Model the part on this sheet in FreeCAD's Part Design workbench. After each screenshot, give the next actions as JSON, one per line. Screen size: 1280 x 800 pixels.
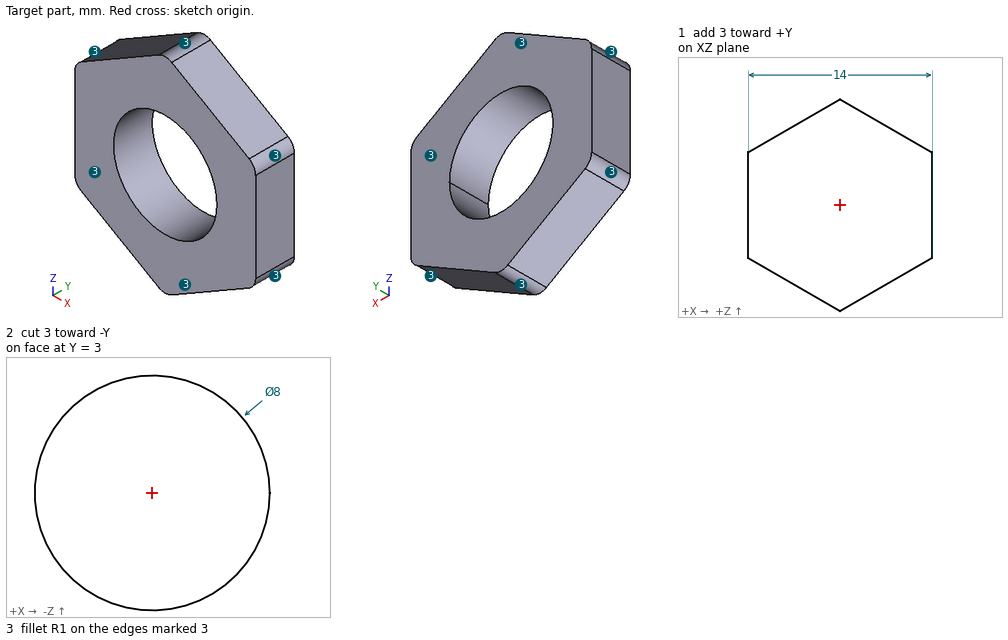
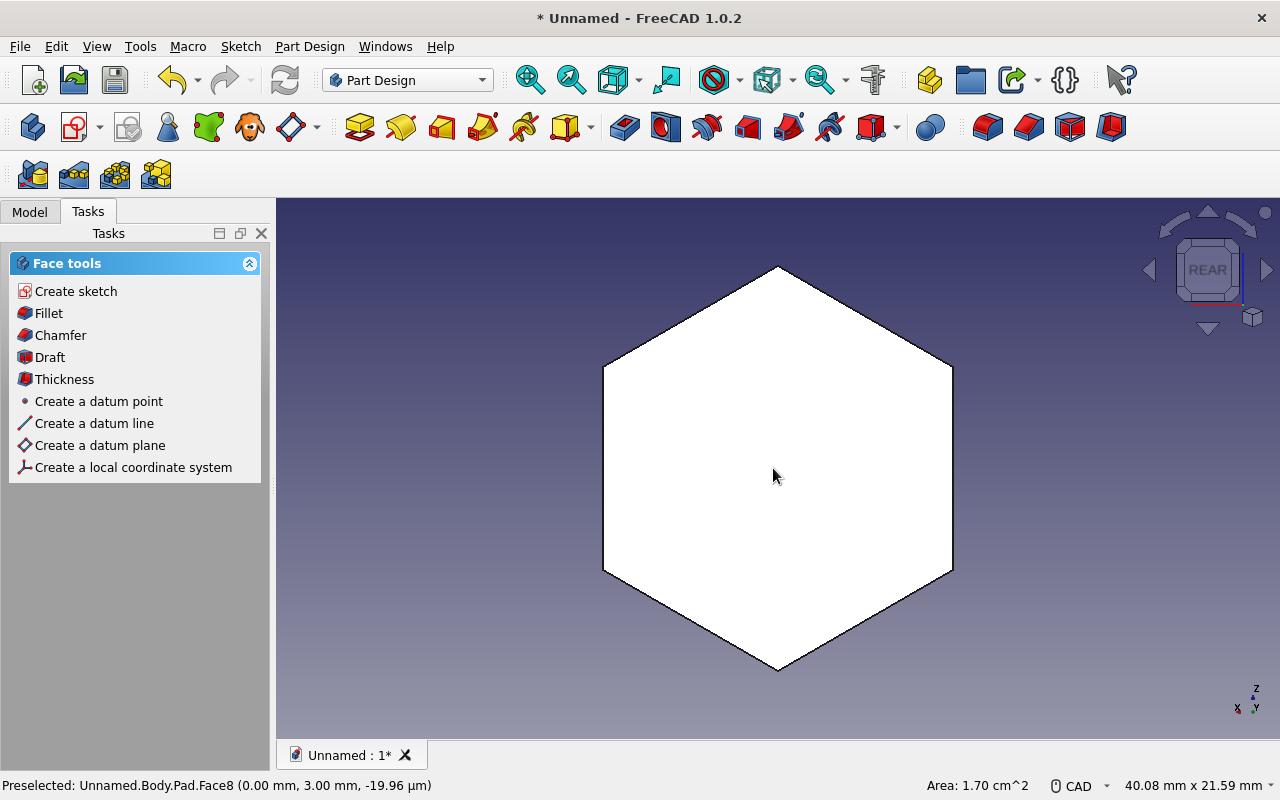
{"action": "left_click", "coordinate": [74, 128]}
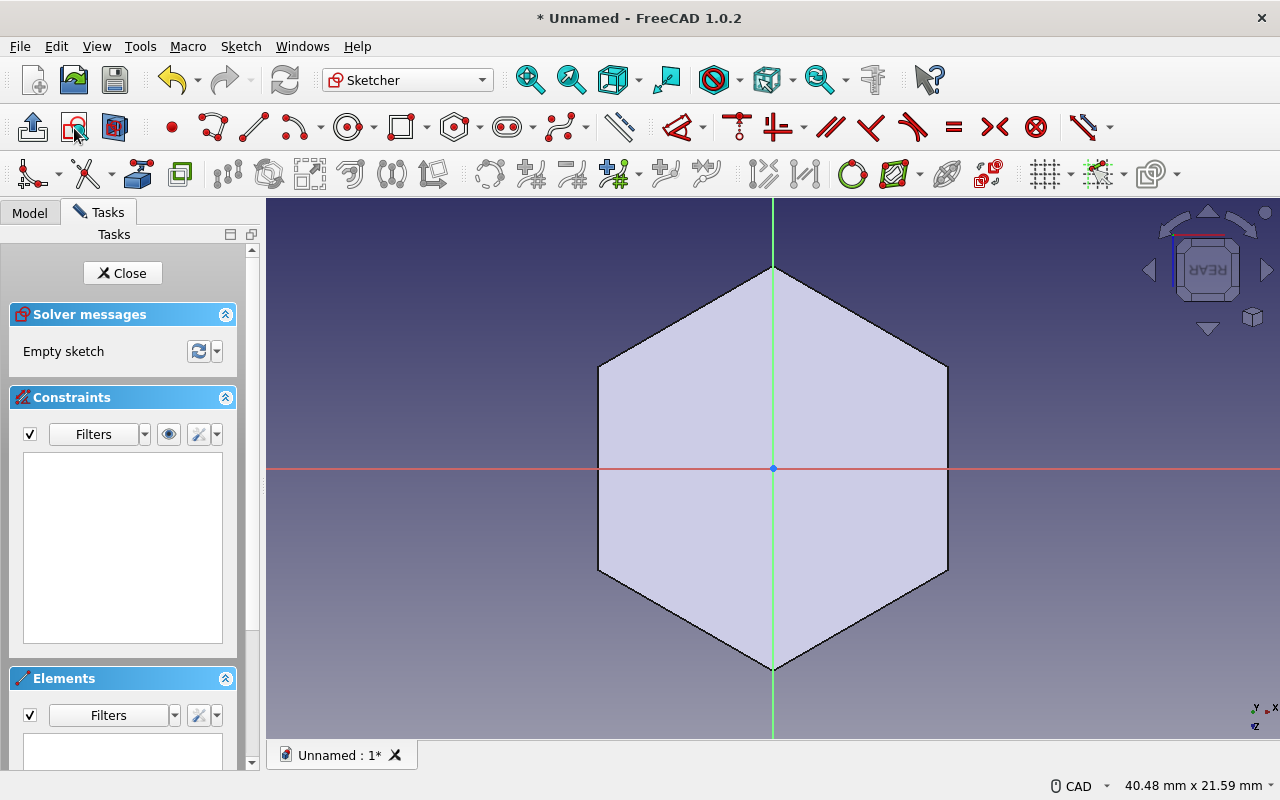
{"action": "scroll", "coordinate": [856, 468], "scroll_direction": "up", "scroll_amount": 3}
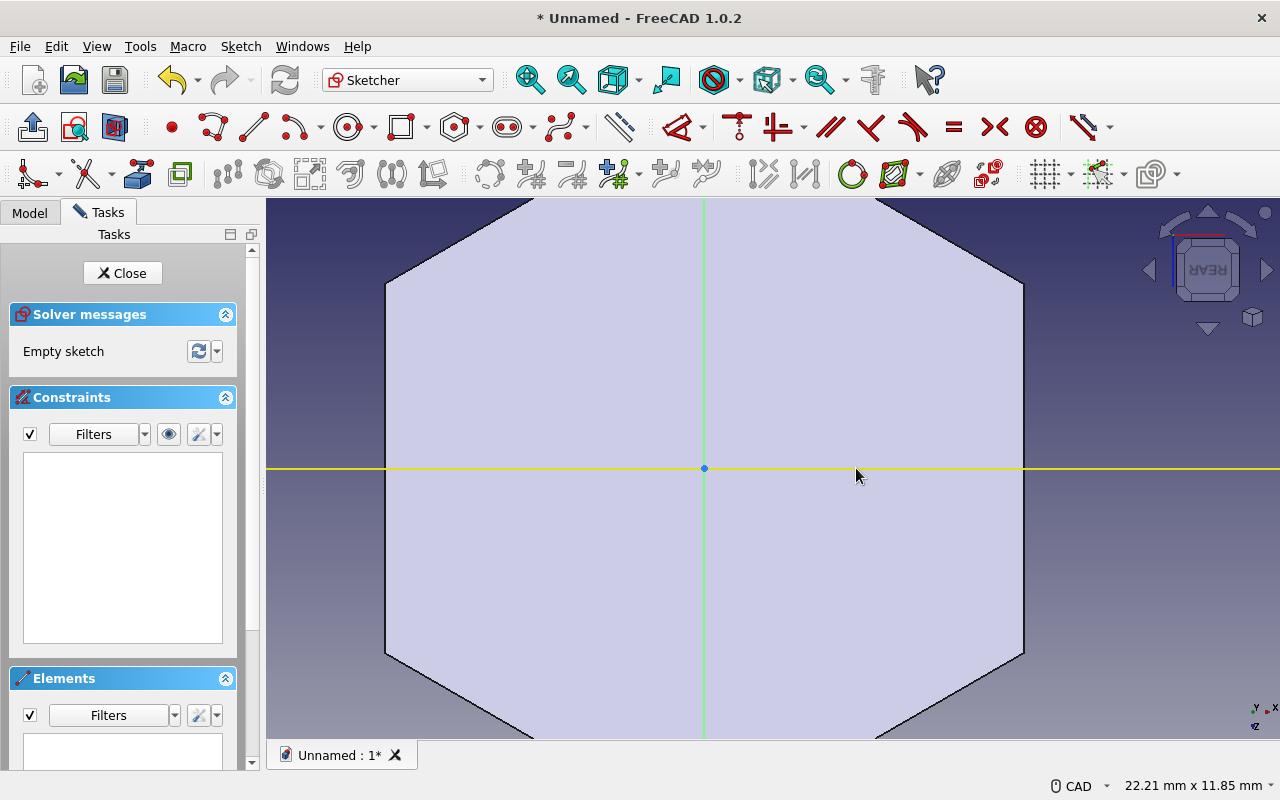
{"action": "key", "text": "g c"}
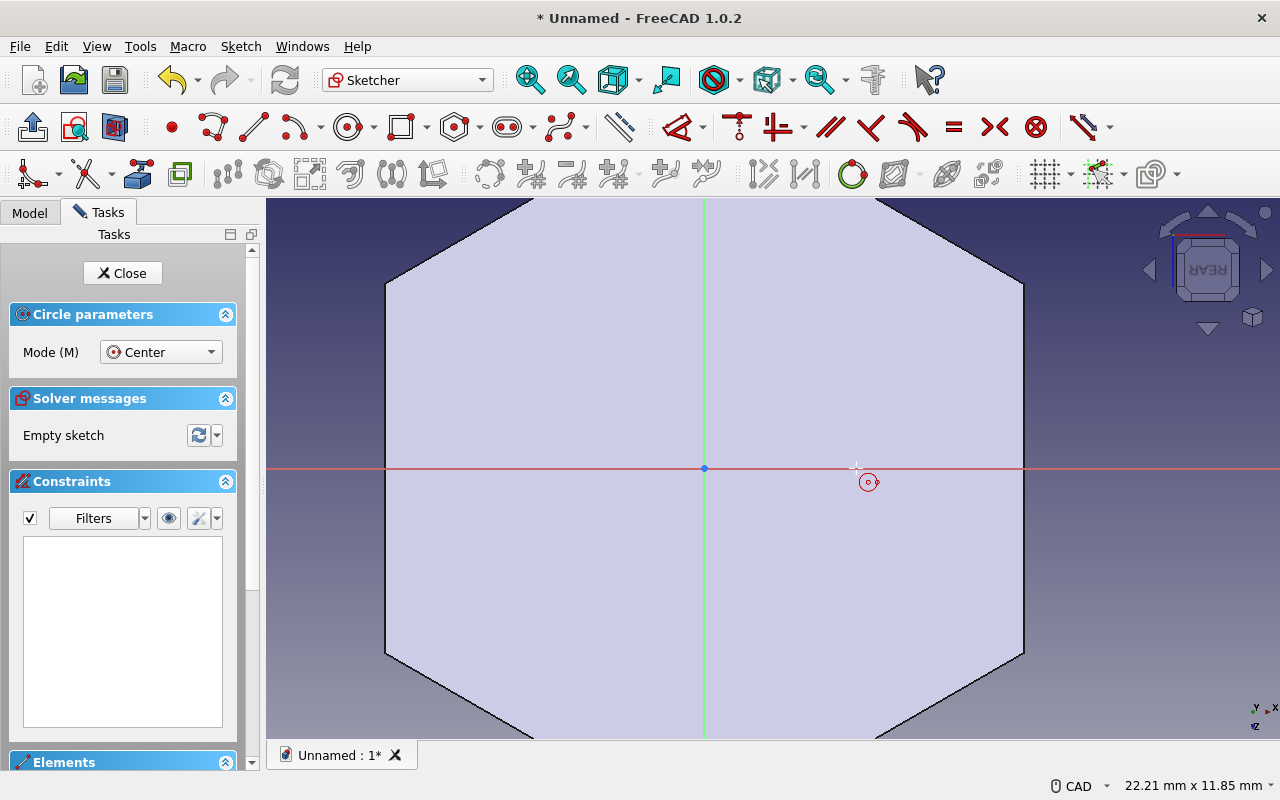
{"action": "left_click", "coordinate": [704, 468]}
{"action": "left_click", "coordinate": [833, 339]}
{"action": "key", "text": "Escape"}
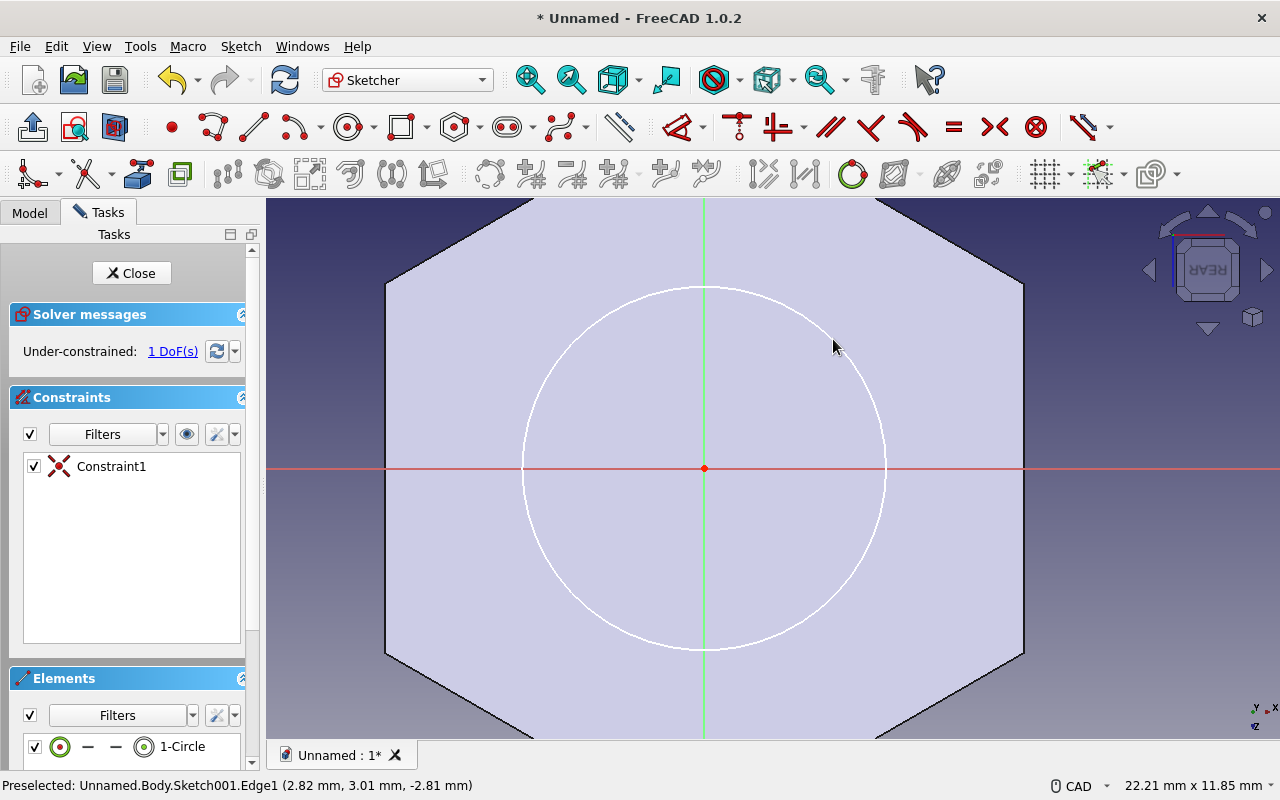
{"action": "key", "text": "d"}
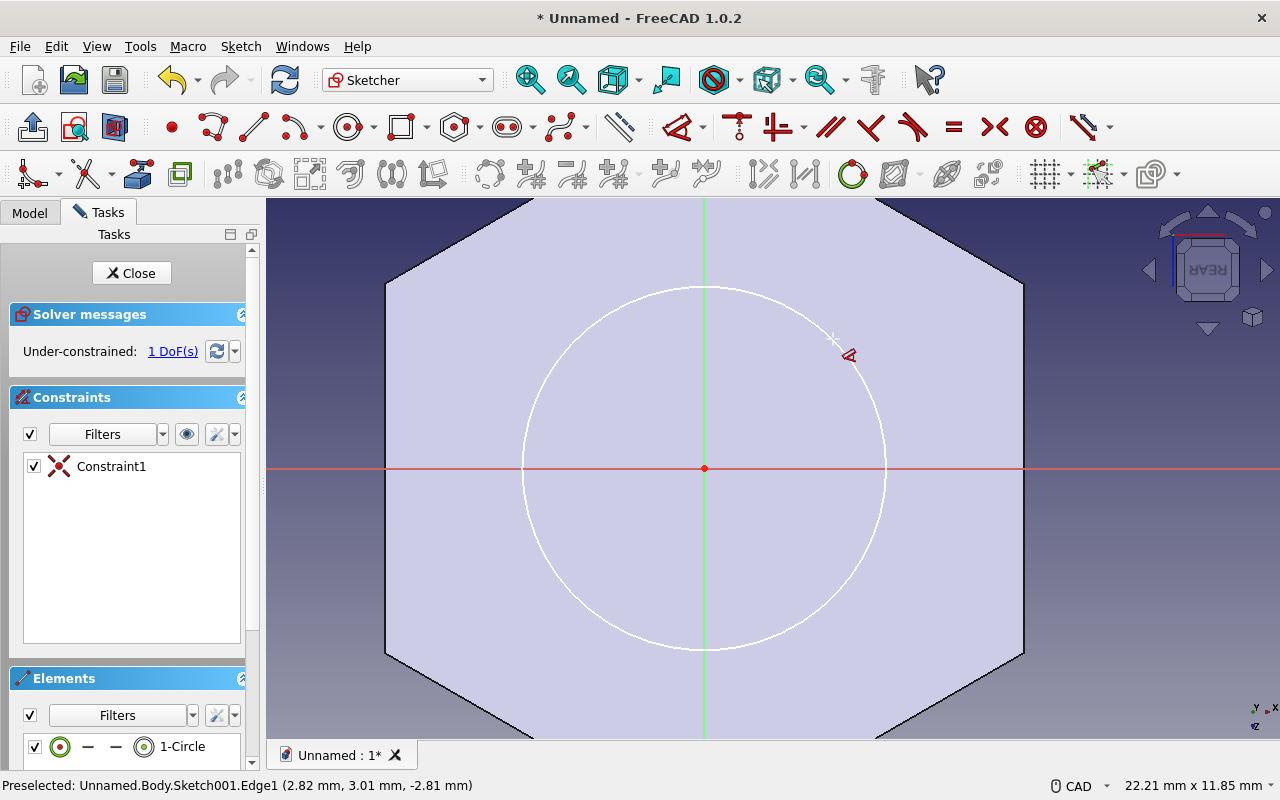
{"action": "left_click", "coordinate": [832, 339]}
{"action": "left_click", "coordinate": [854, 316]}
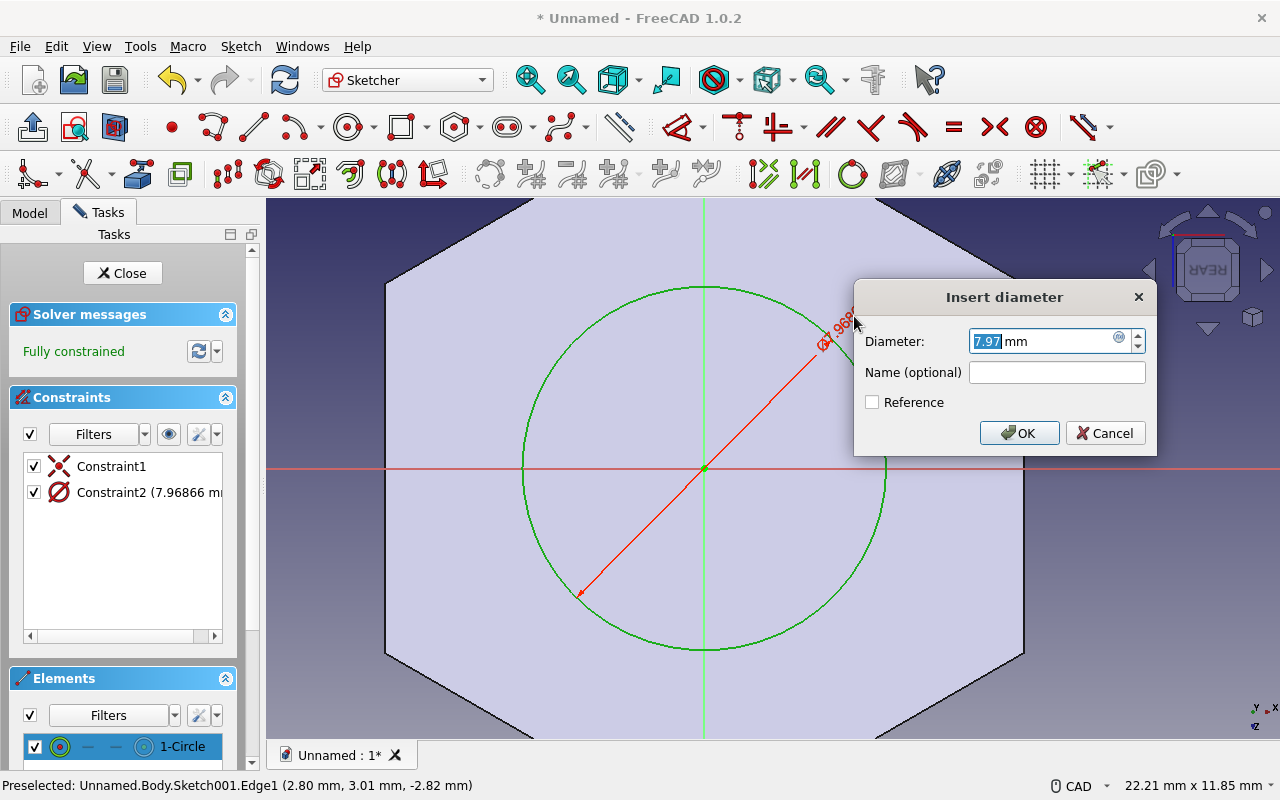
{"action": "type", "text": "8"}
{"action": "key", "text": "Return"}
{"action": "key", "text": "Escape"}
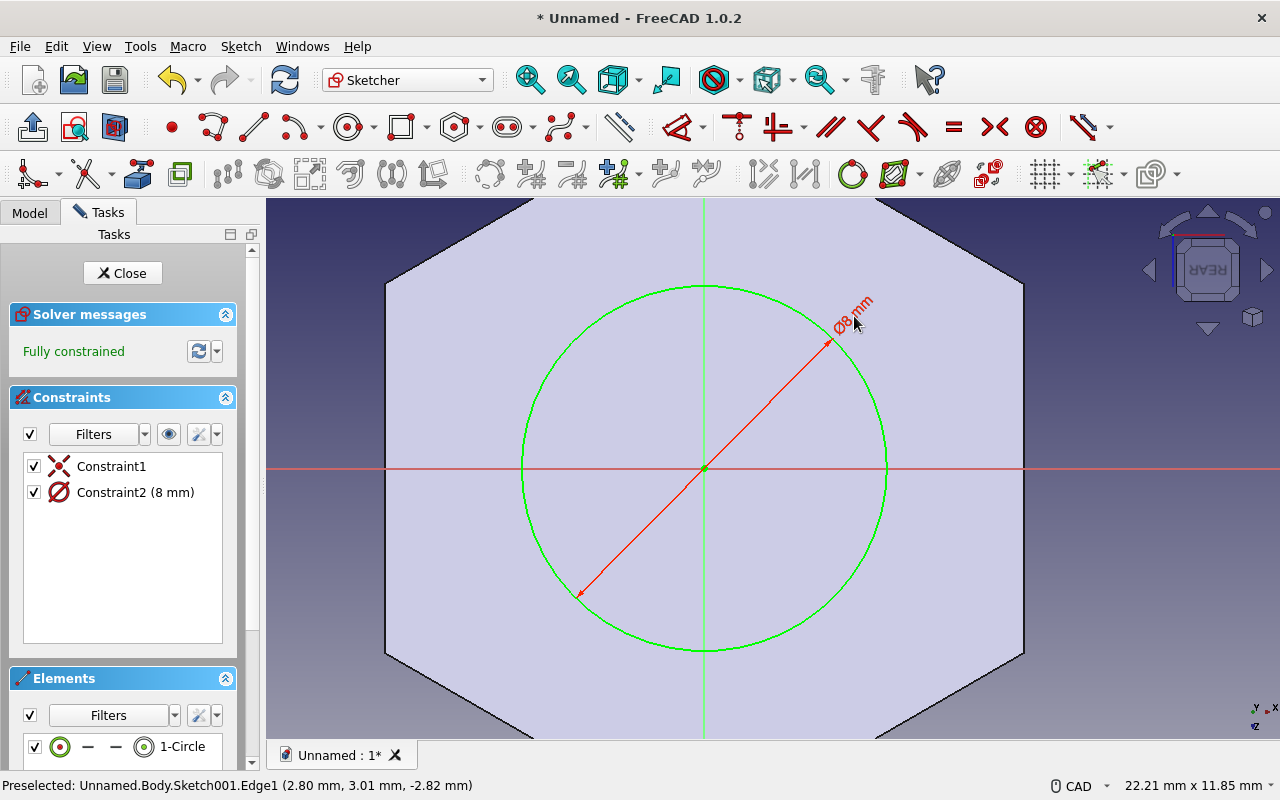
{"action": "left_click", "coordinate": [123, 273]}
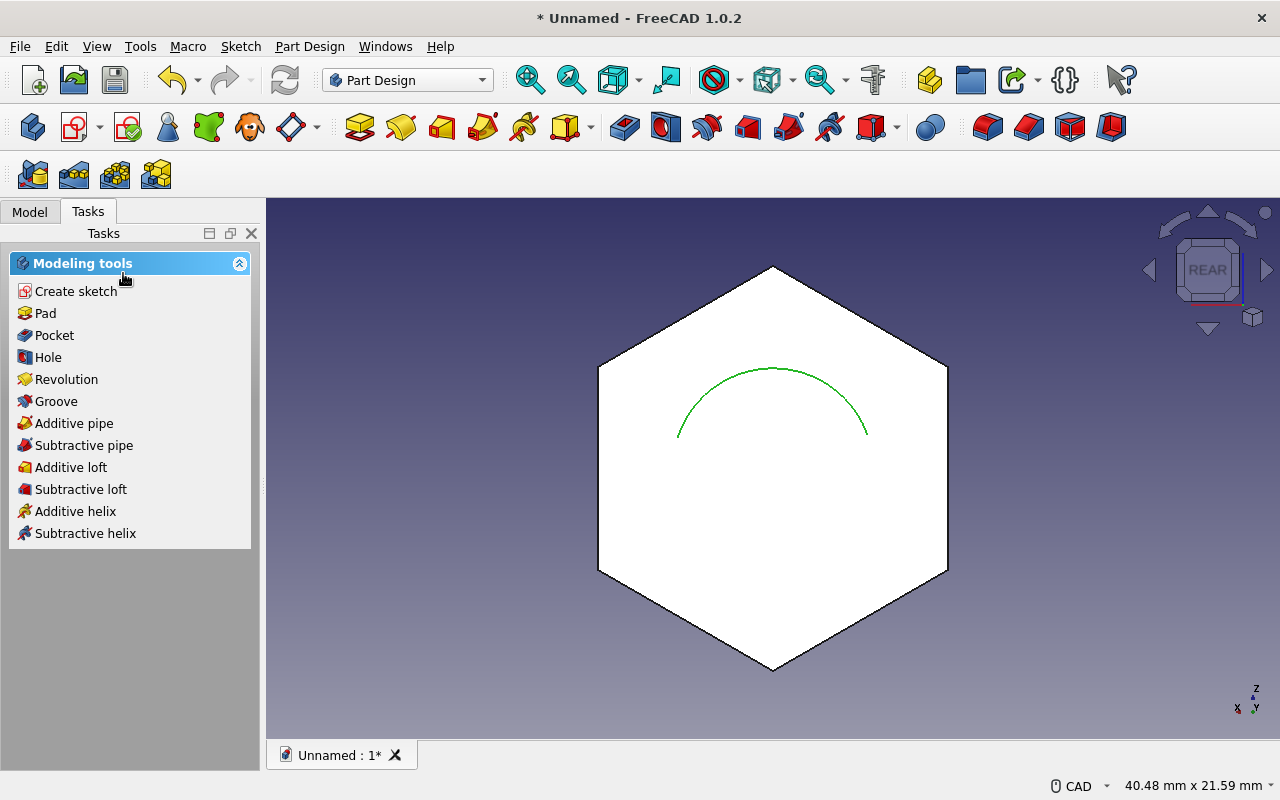
{"action": "left_click", "coordinate": [625, 128]}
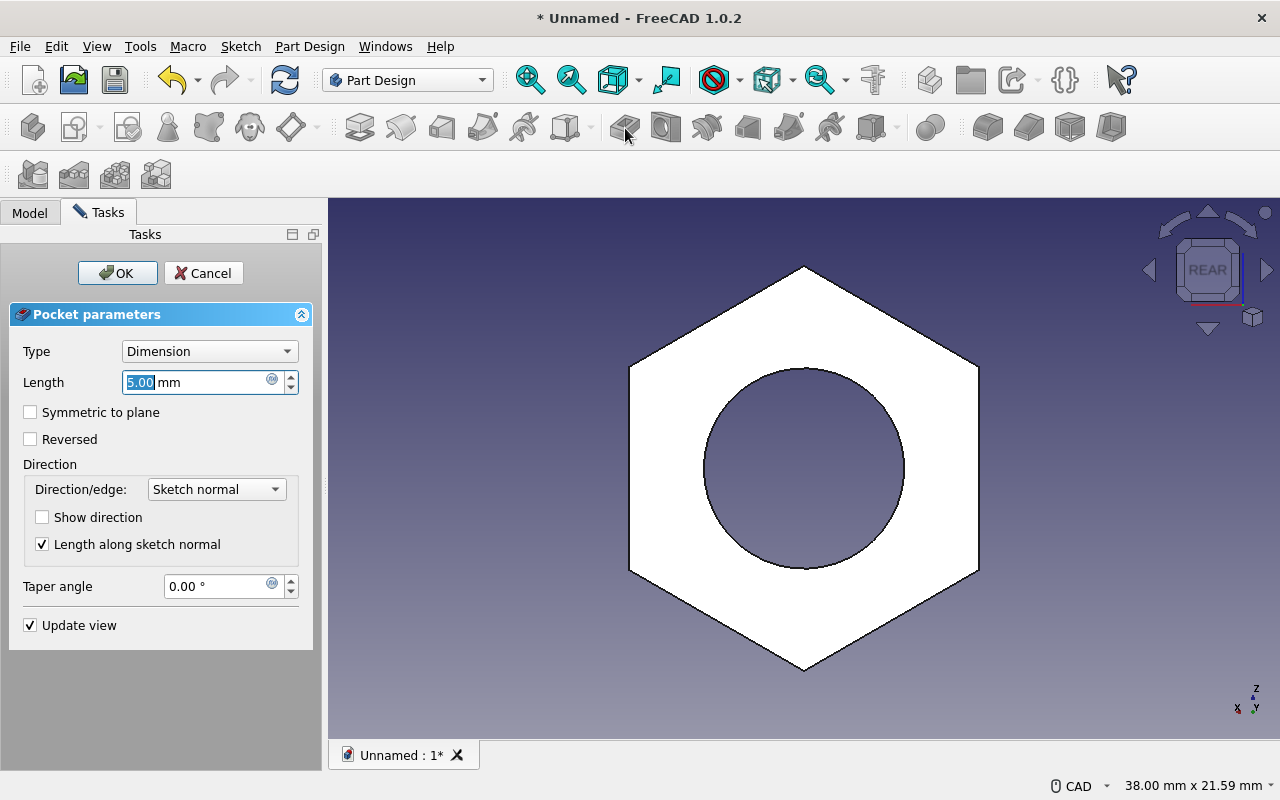
{"action": "type", "text": "3"}
{"action": "key", "text": "Tab"}